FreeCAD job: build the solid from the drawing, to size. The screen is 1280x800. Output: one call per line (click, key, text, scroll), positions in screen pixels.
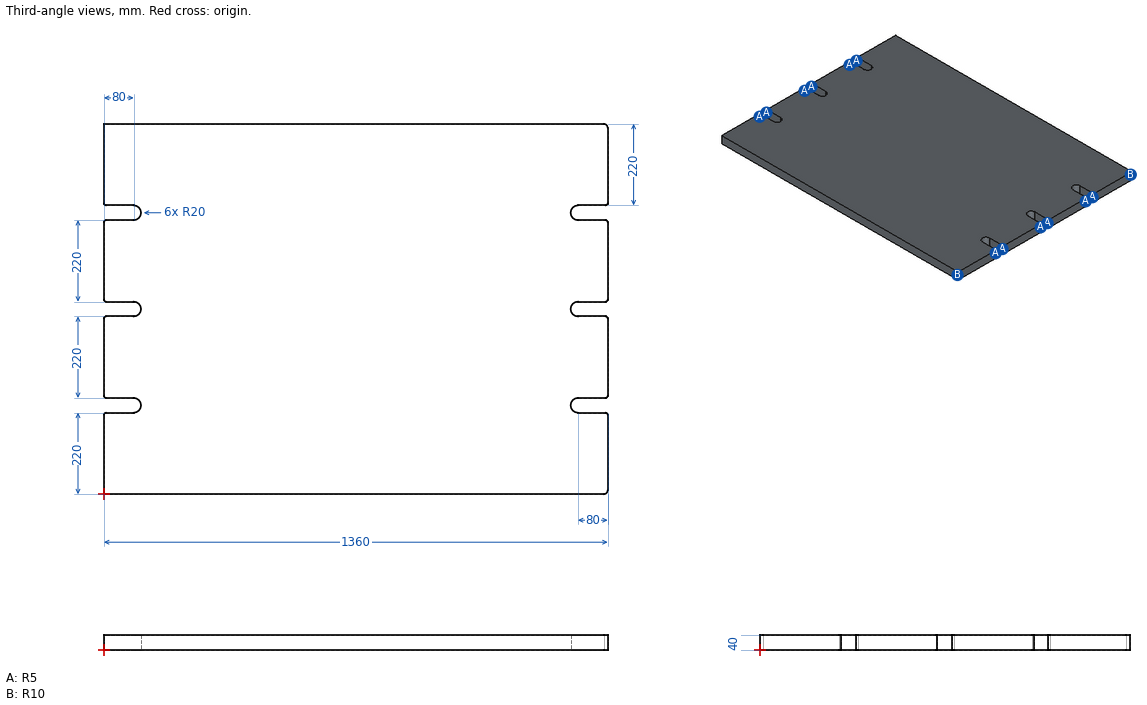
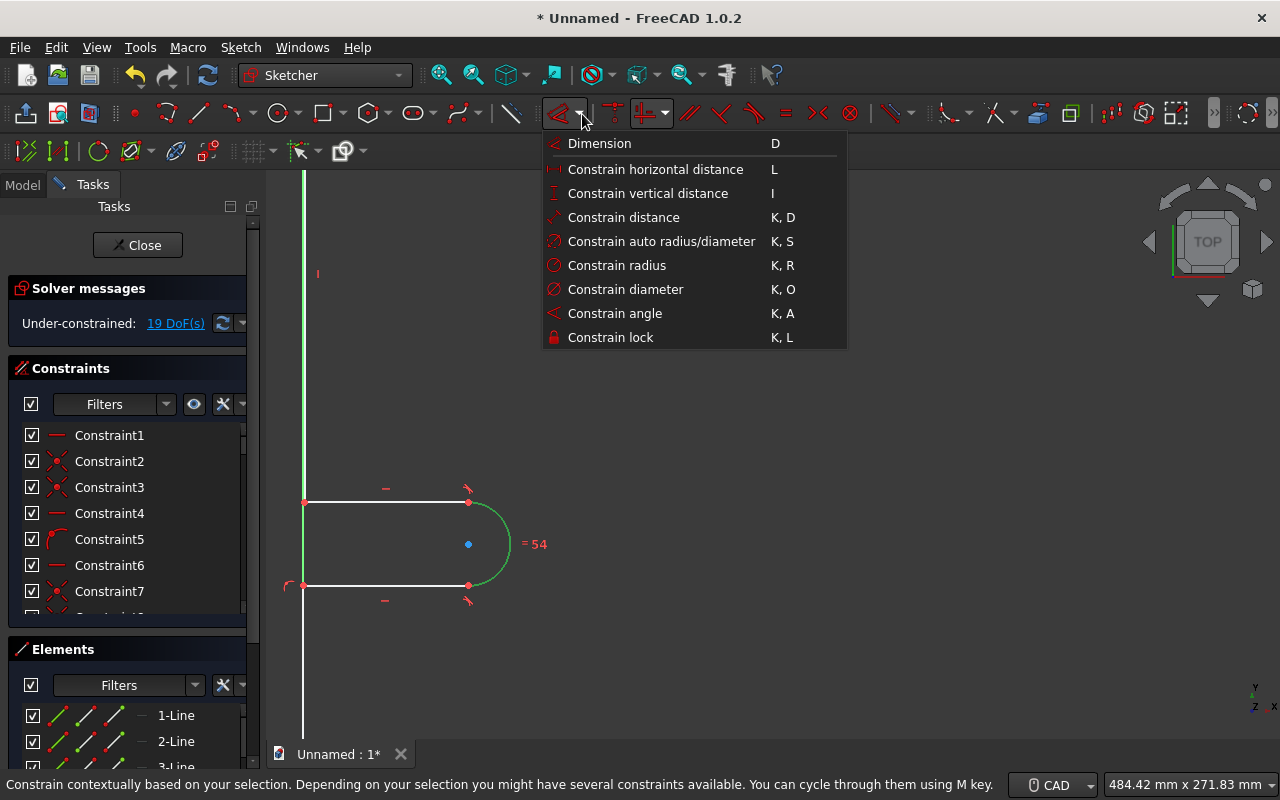
click(695, 265)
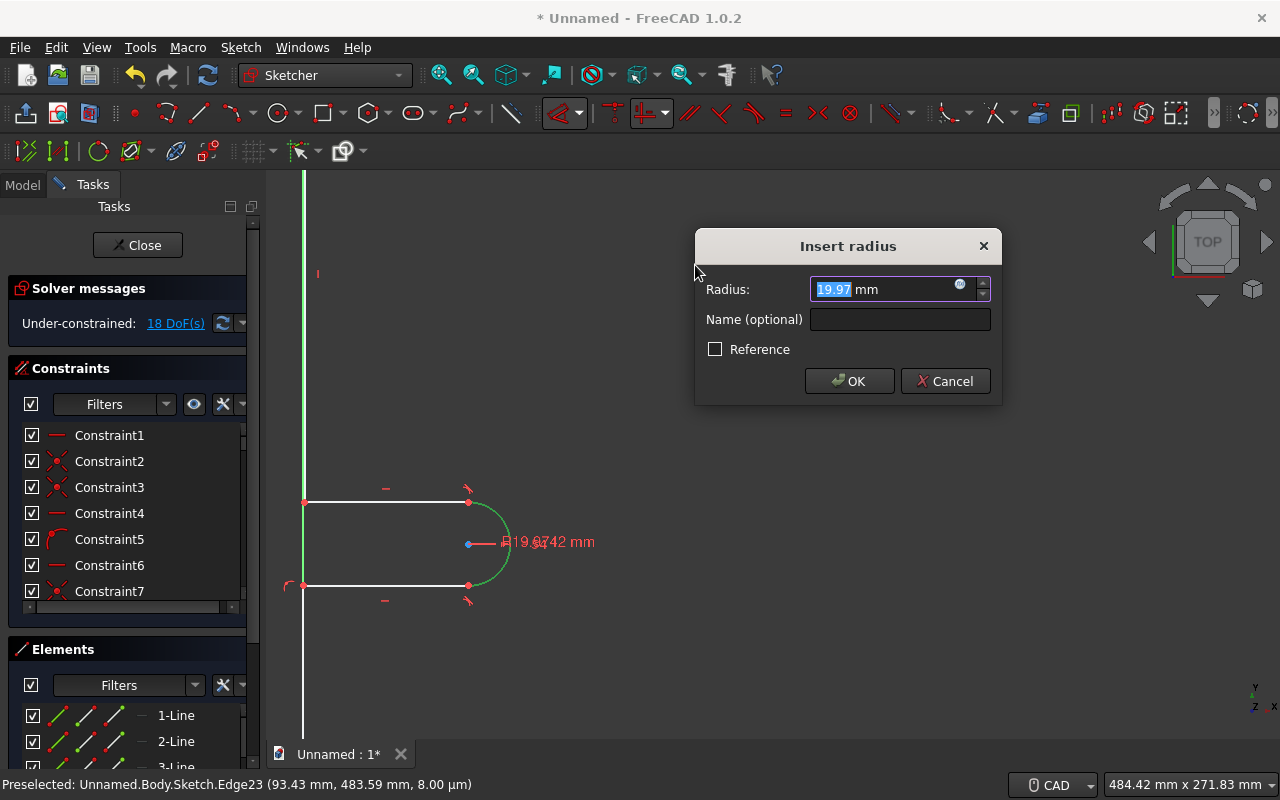
text(20)
key(Return)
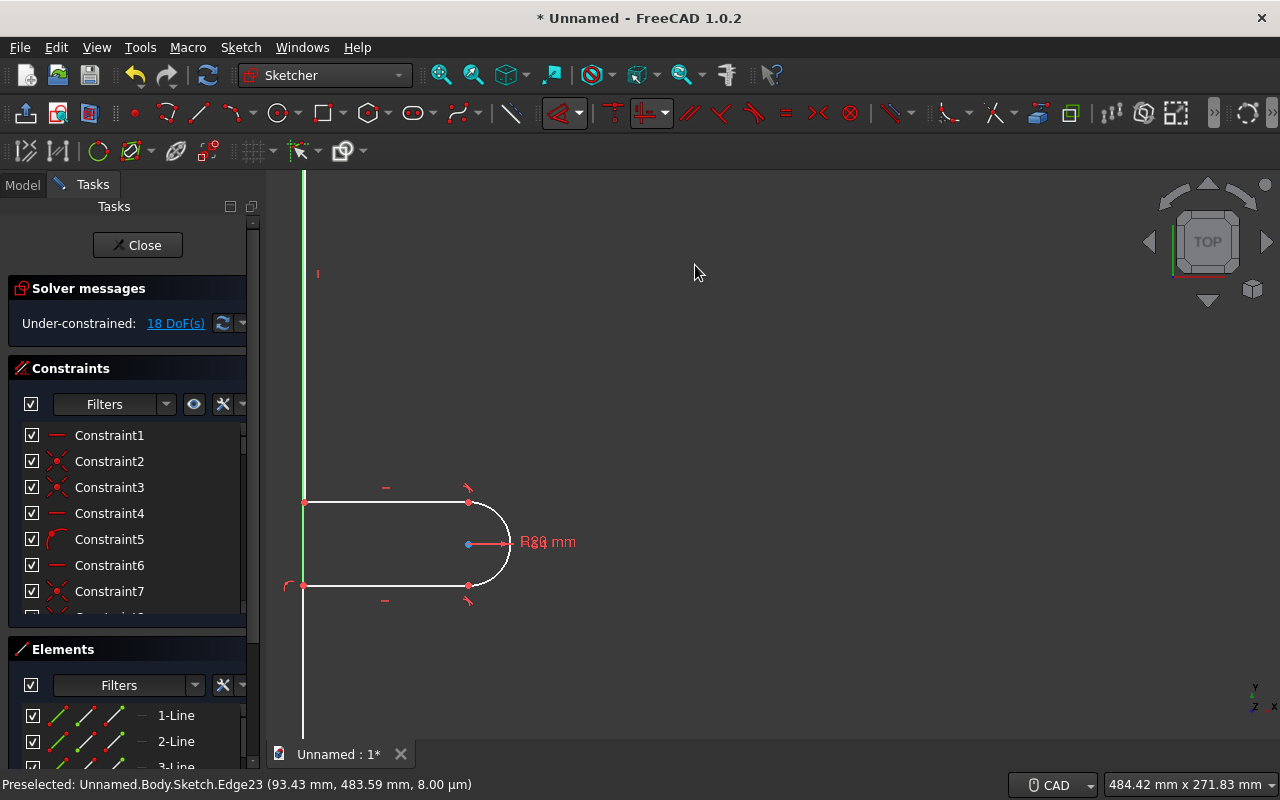
scroll(502, 438, down, 9)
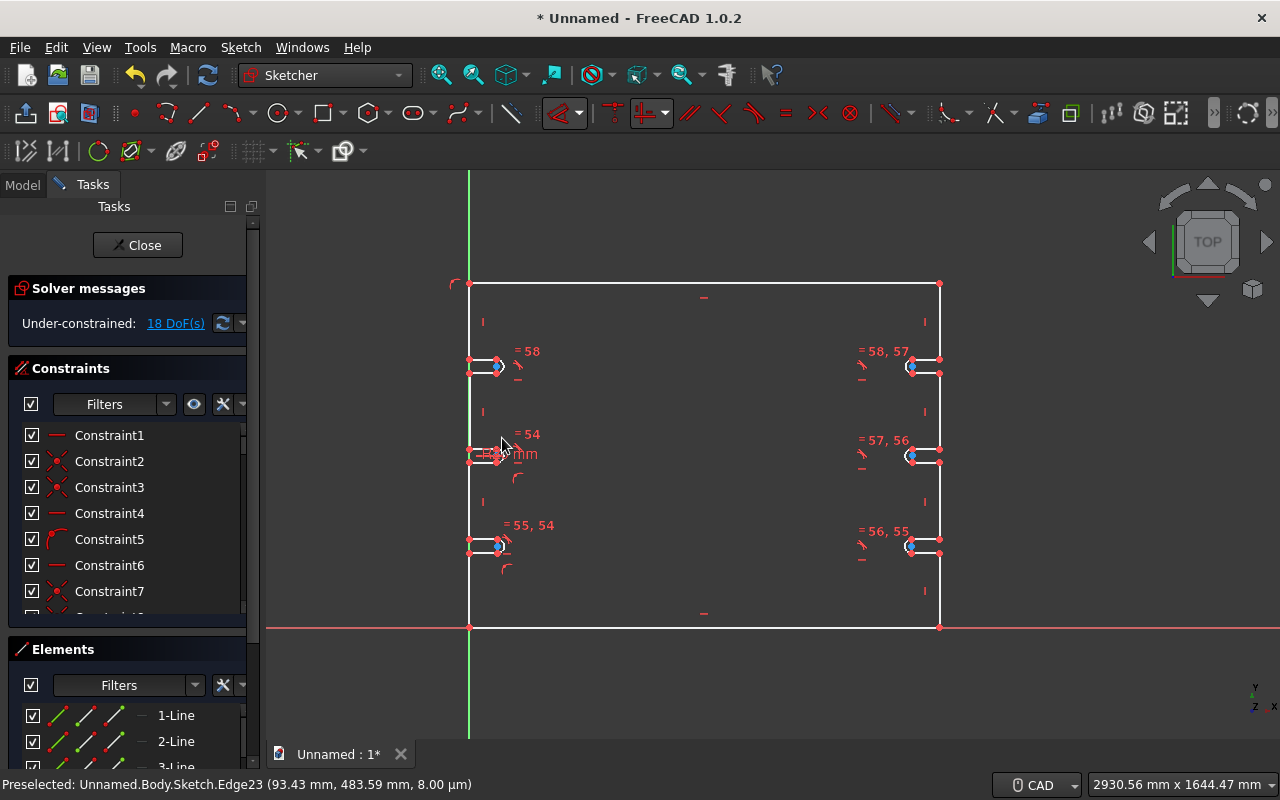
click(470, 373)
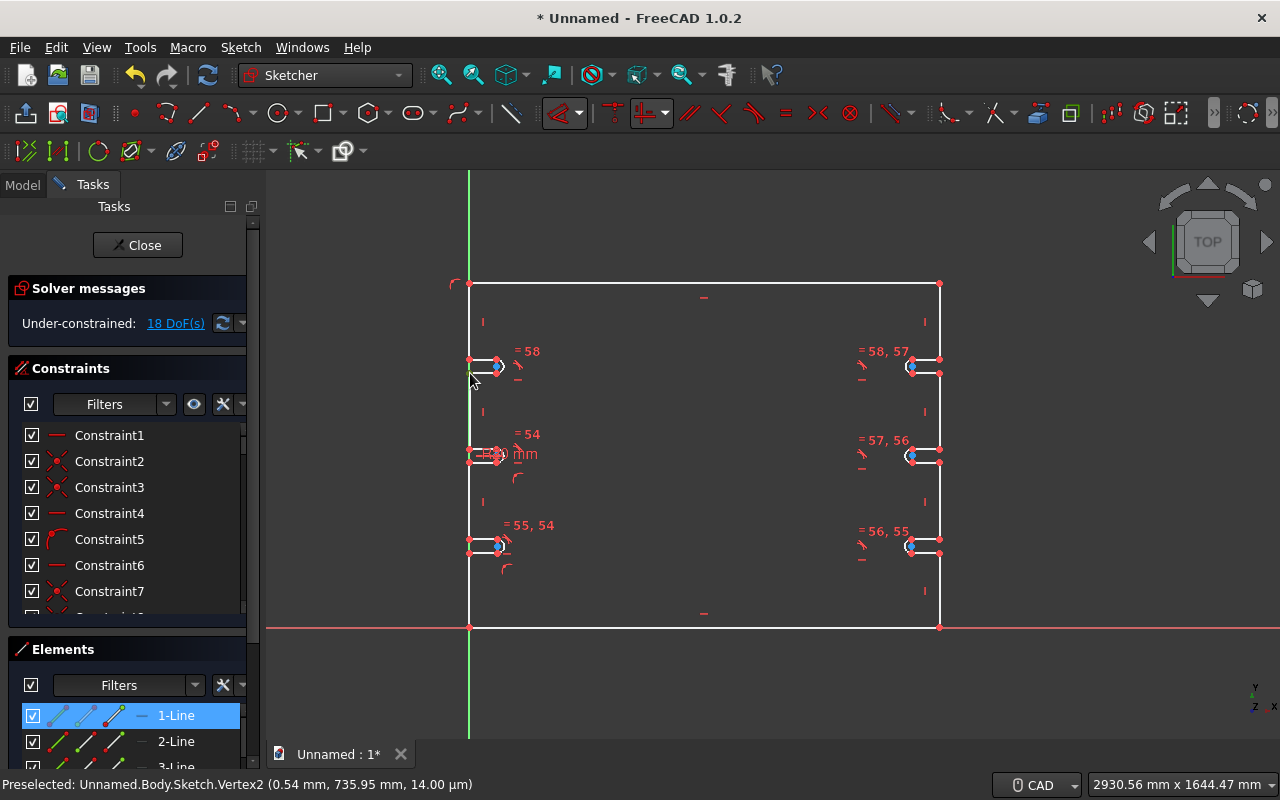
click(469, 674)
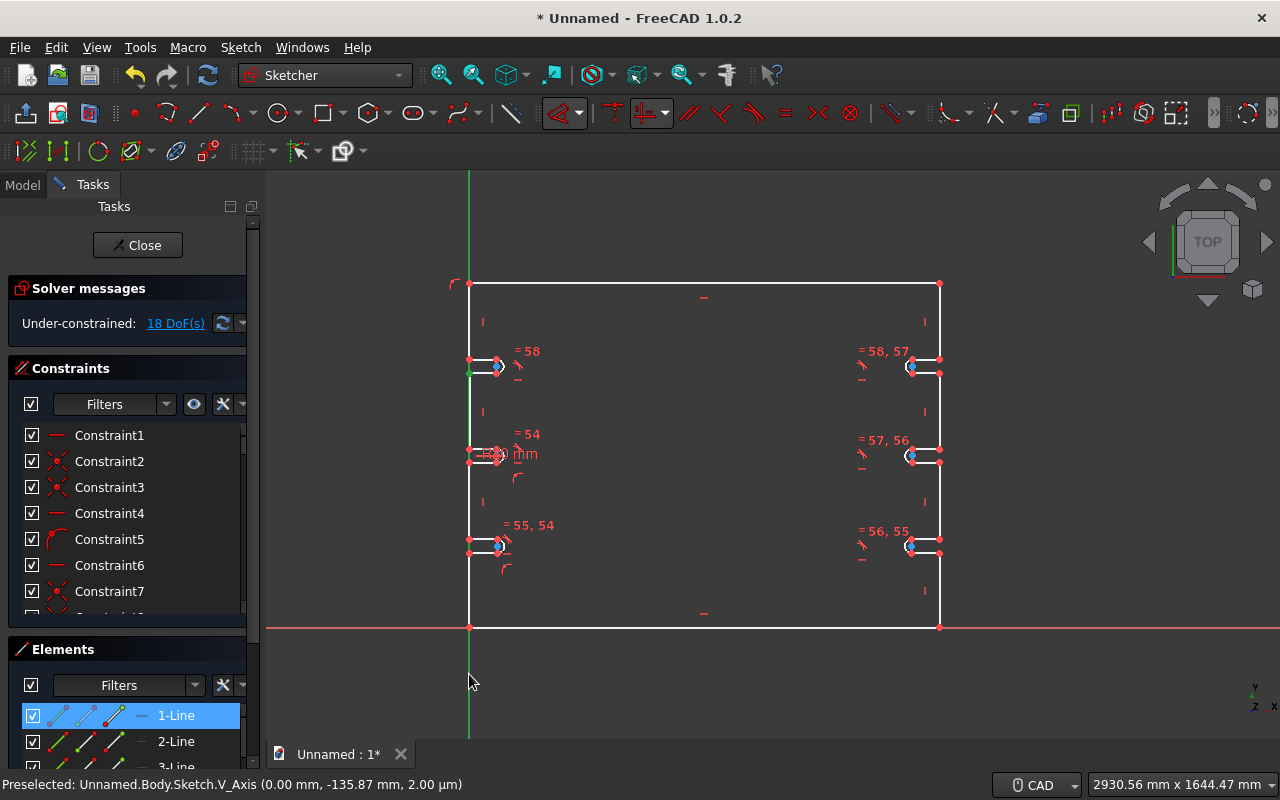
click(614, 114)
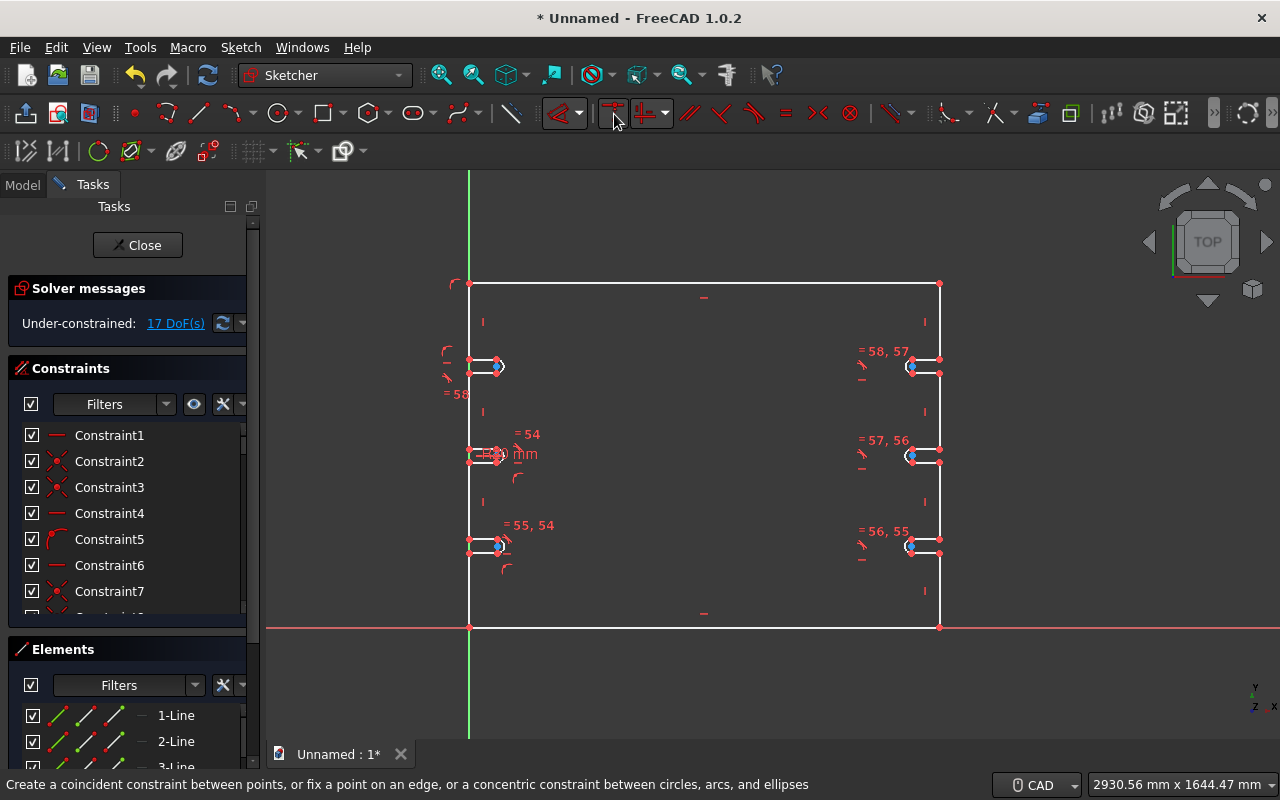
scroll(486, 373, up, 2)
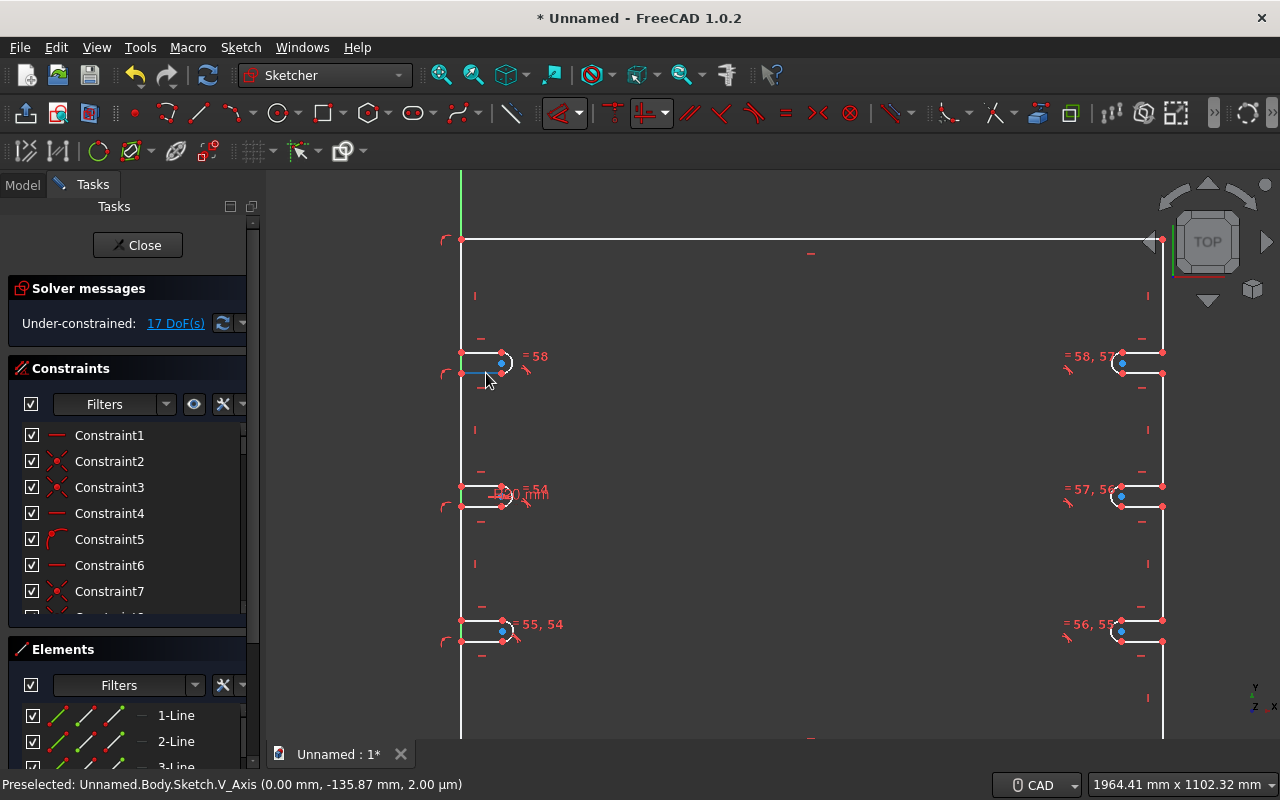
click(486, 373)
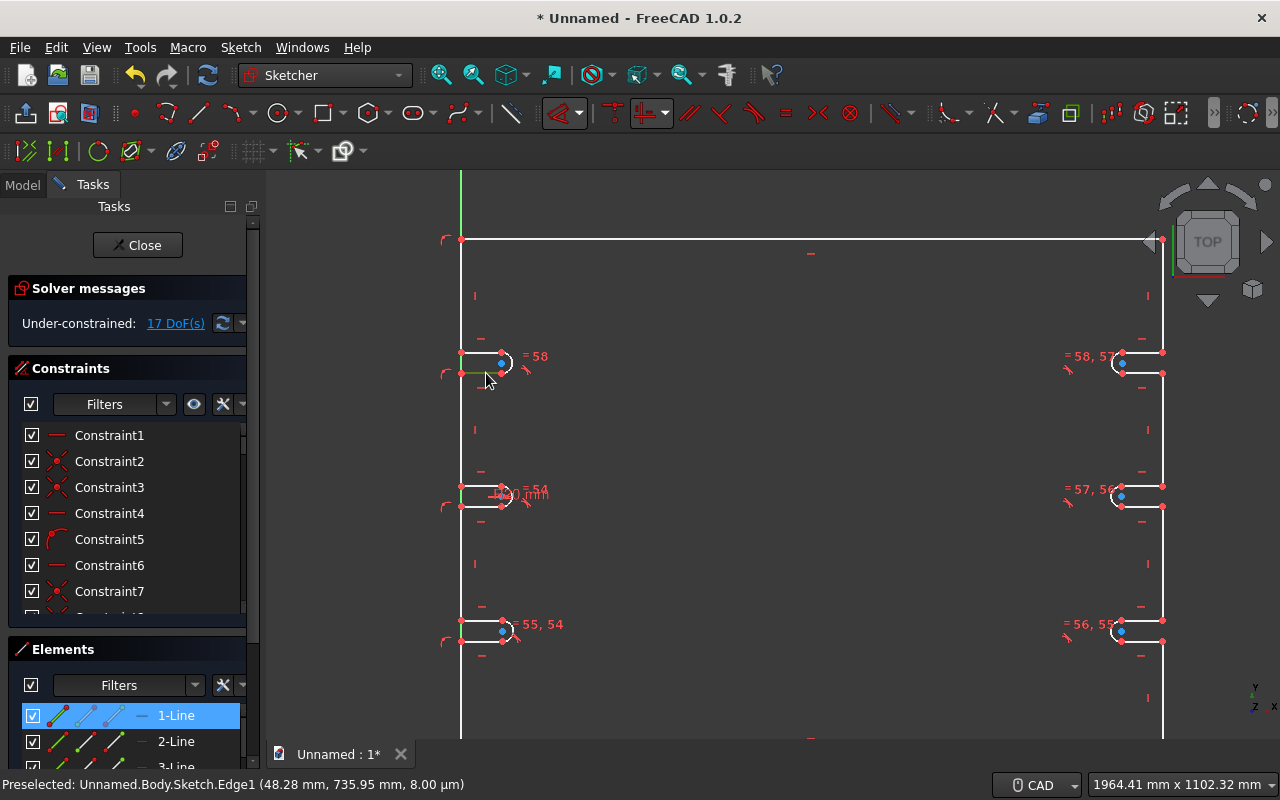
key(l)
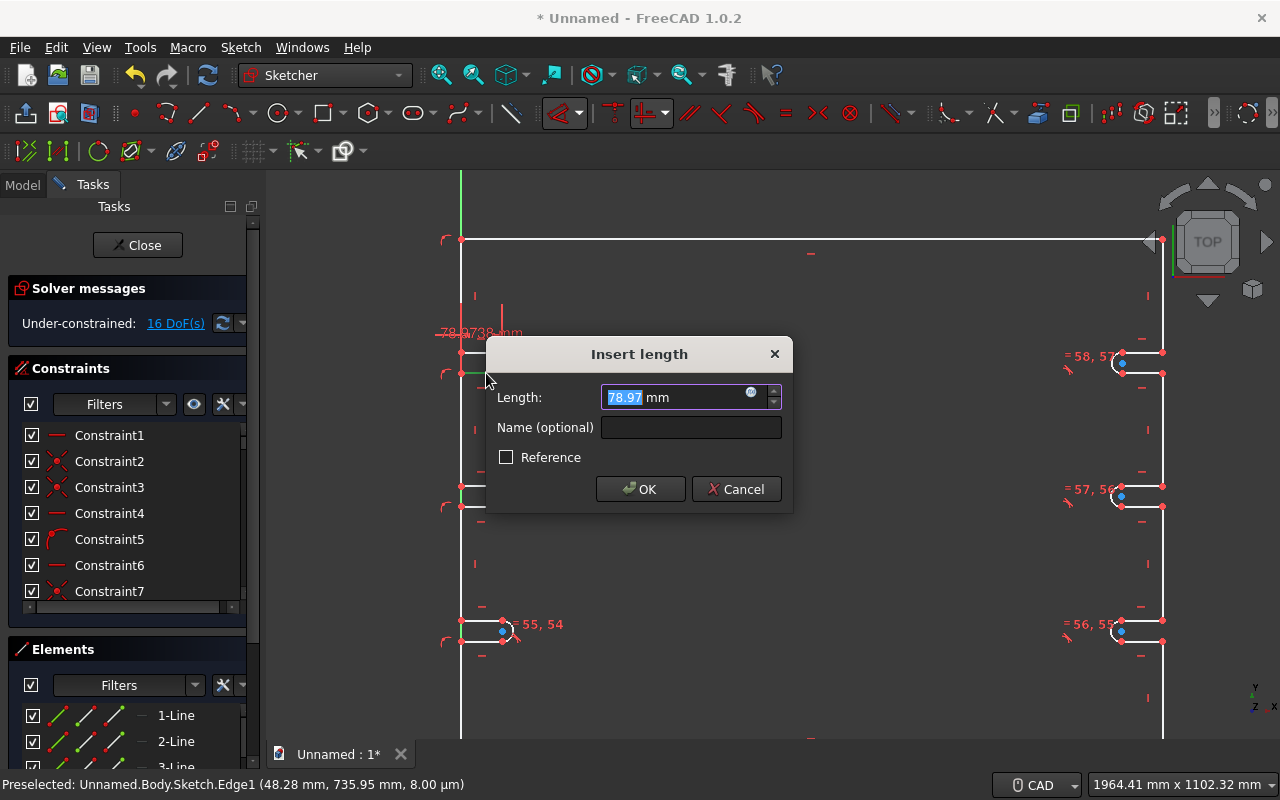
text(80)
key(Return)